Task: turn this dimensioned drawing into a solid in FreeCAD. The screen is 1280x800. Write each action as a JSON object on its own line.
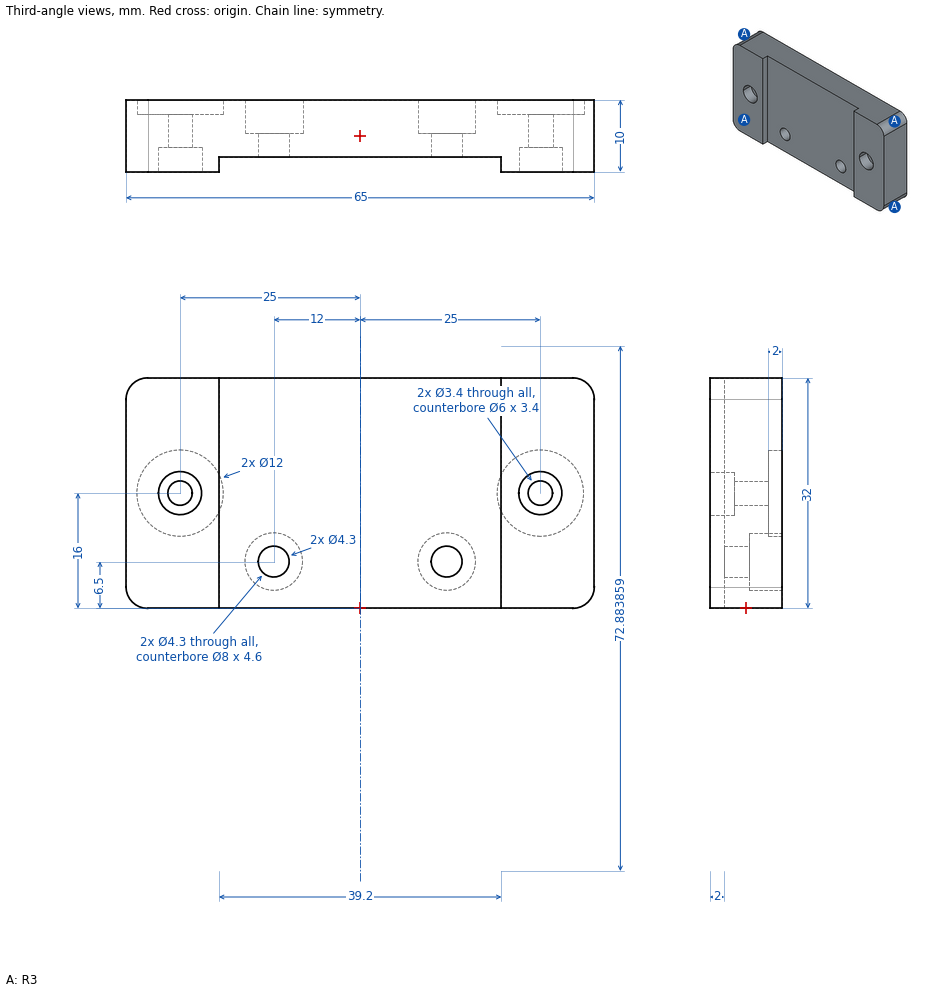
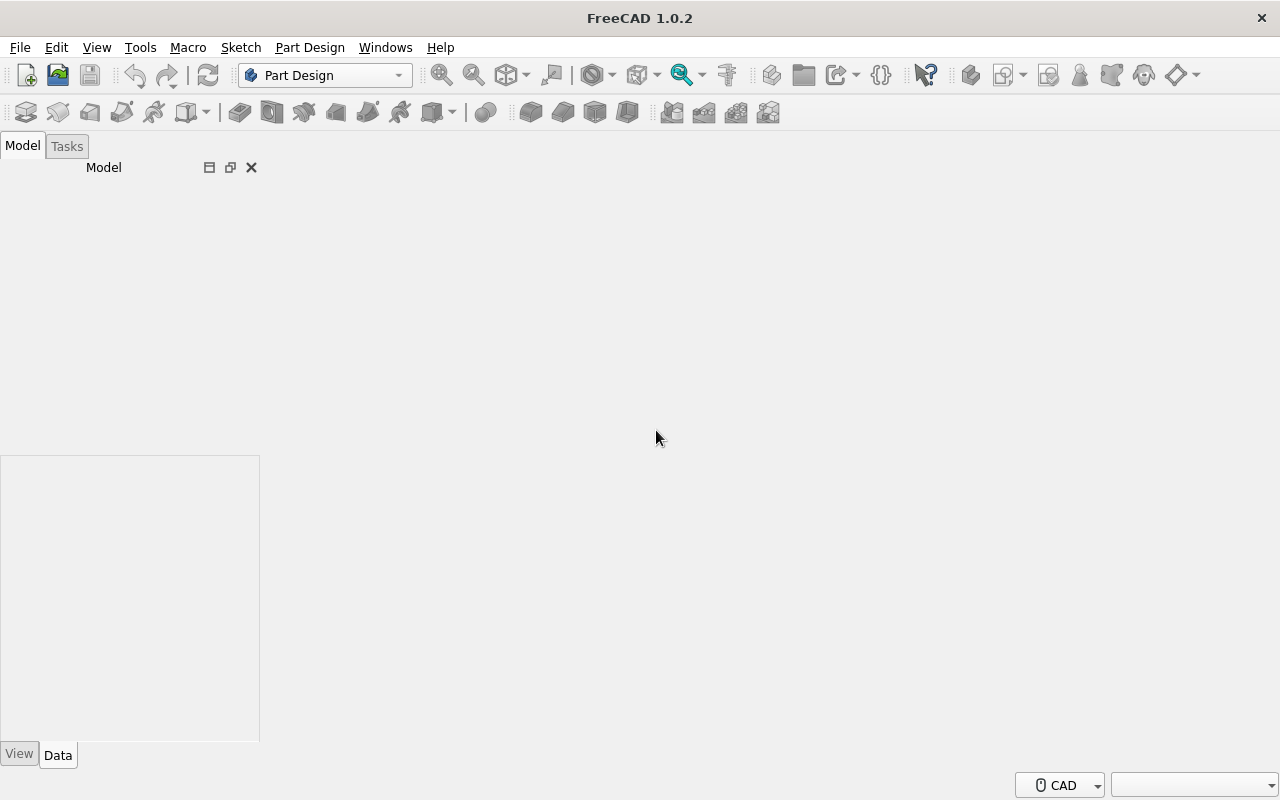
{"action": "left_click", "coordinate": [26, 76]}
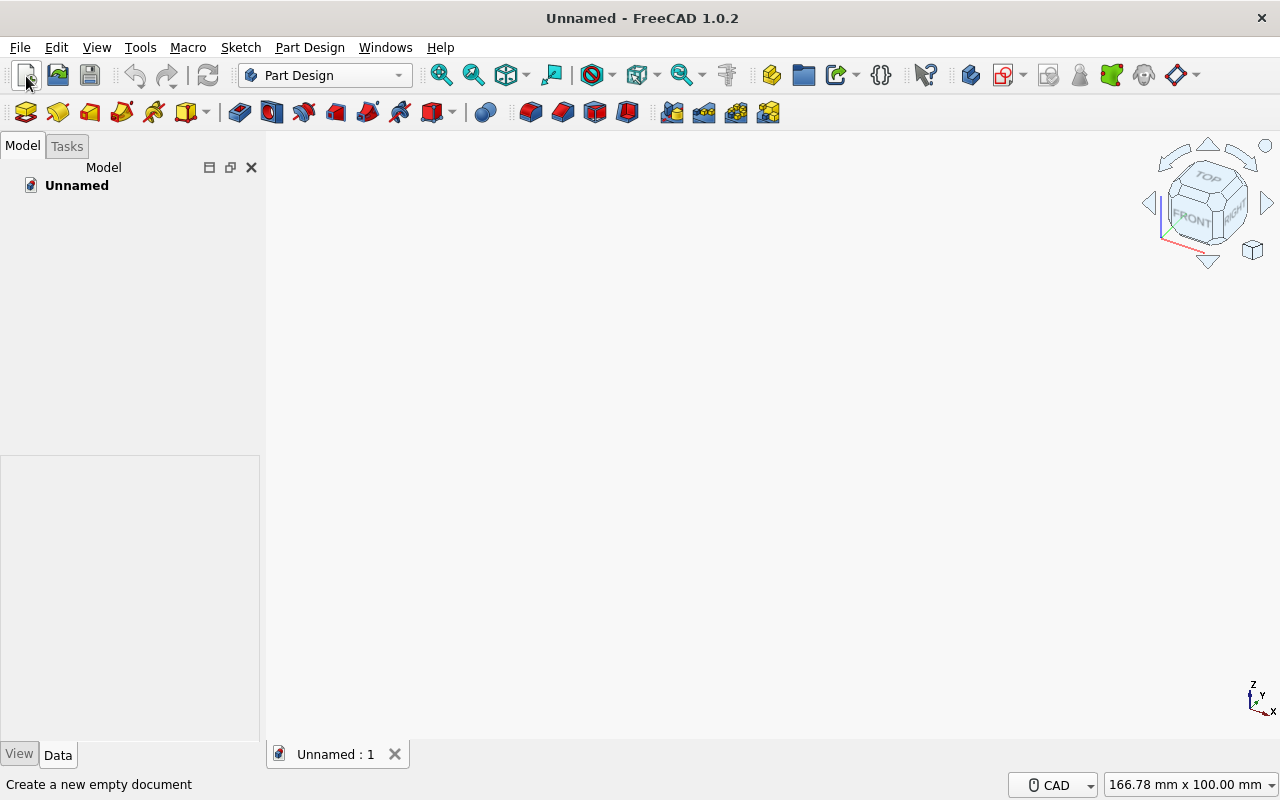
{"action": "left_click", "coordinate": [1004, 76]}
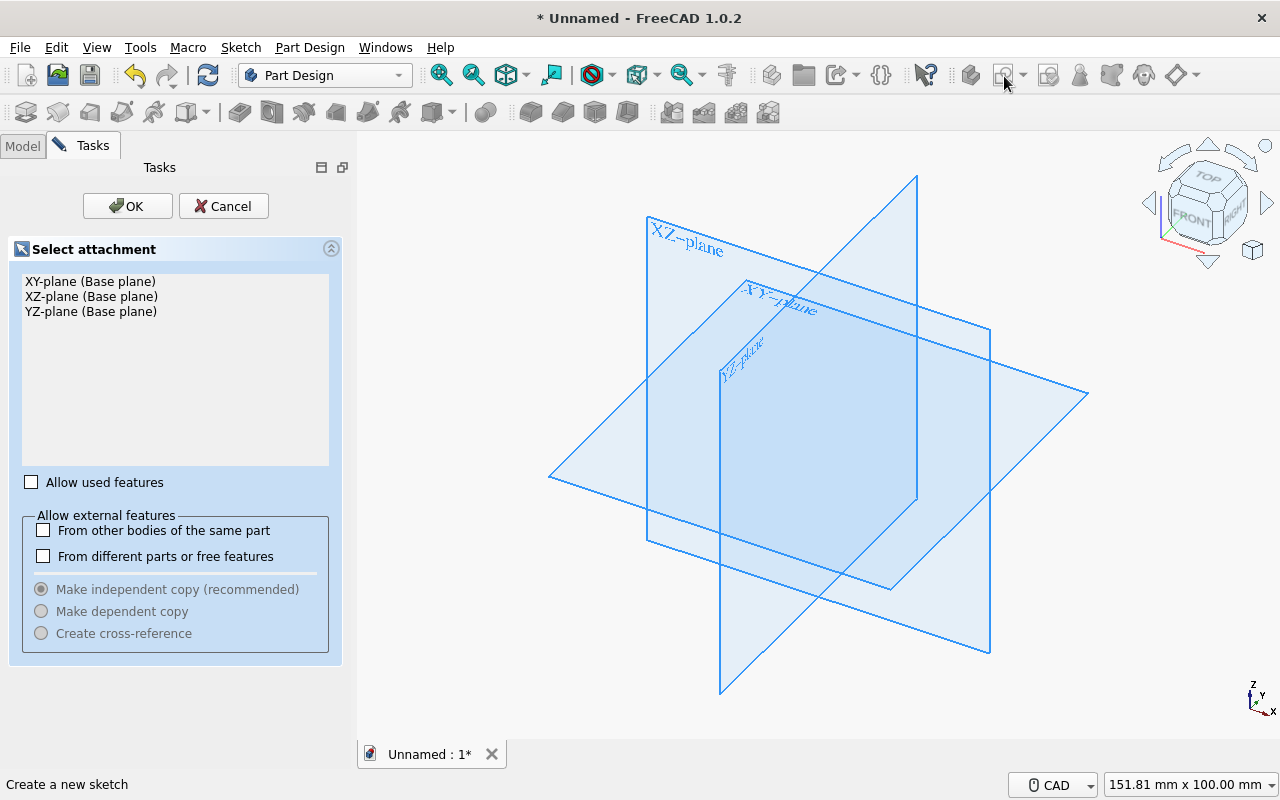
{"action": "left_click", "coordinate": [82, 282]}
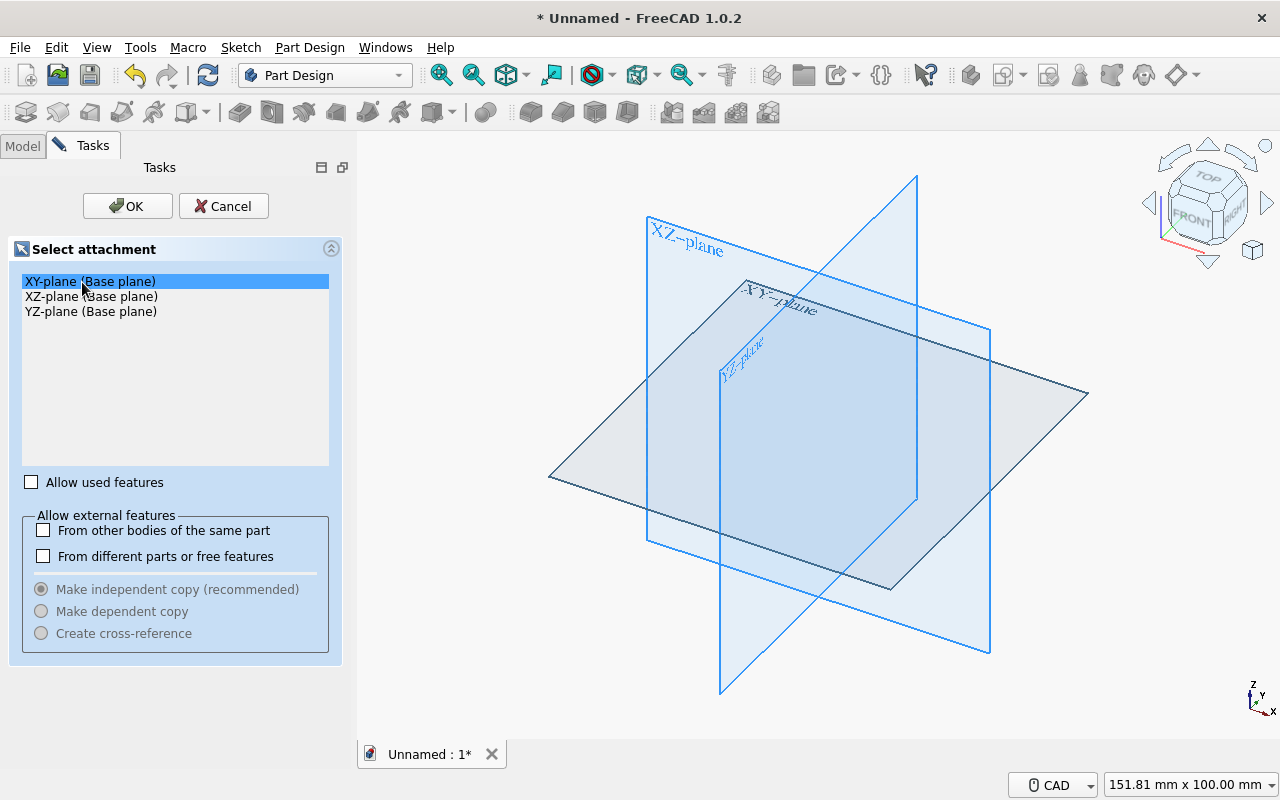
{"action": "left_click", "coordinate": [128, 206]}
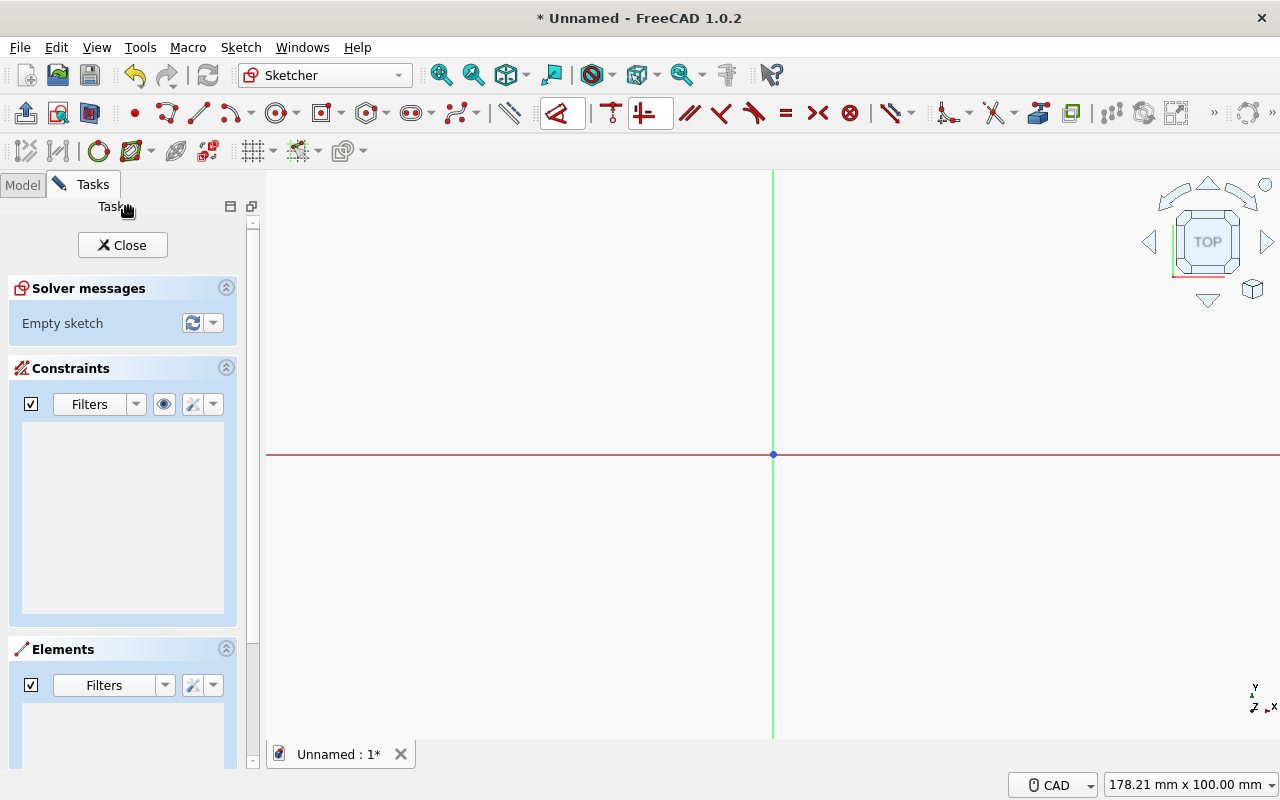
{"action": "scroll", "coordinate": [912, 455], "scroll_direction": "up", "scroll_amount": 2}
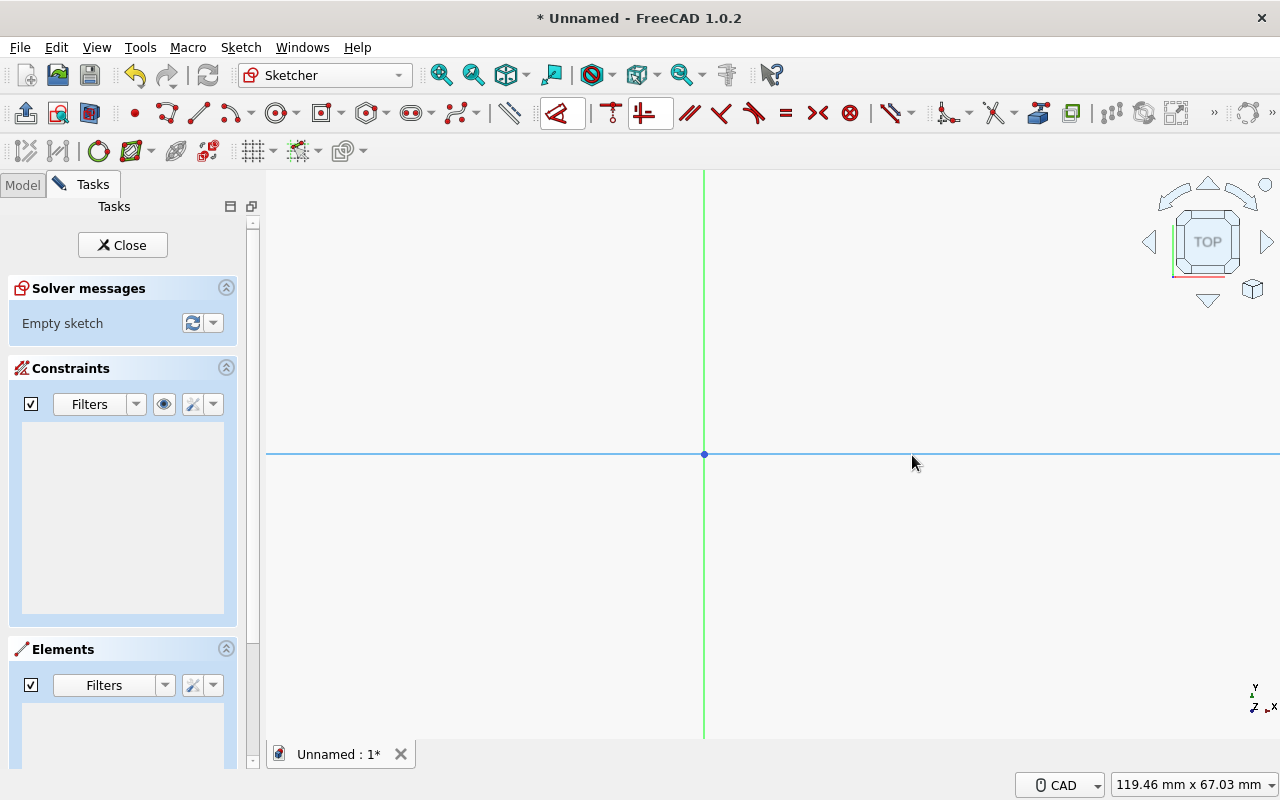
{"action": "left_click", "coordinate": [322, 114]}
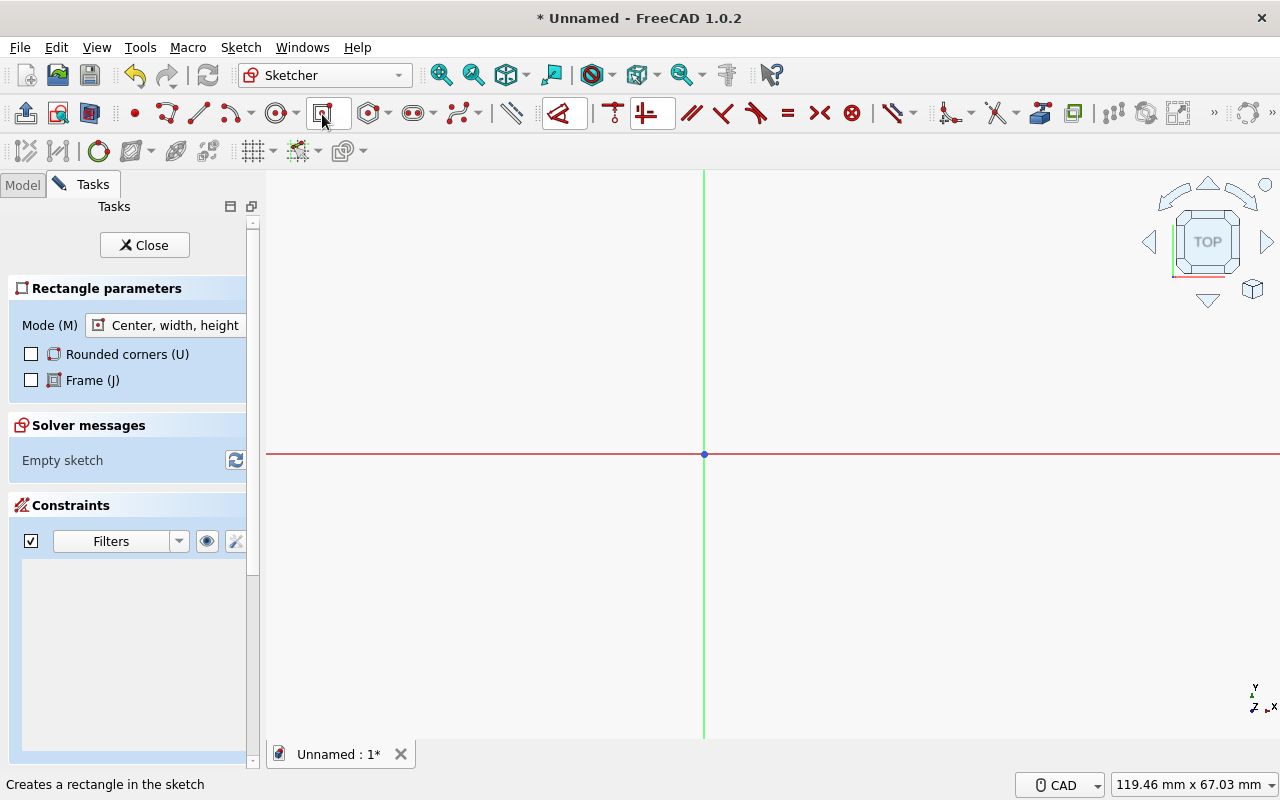
{"action": "left_click", "coordinate": [704, 454]}
{"action": "left_click", "coordinate": [980, 412]}
{"action": "key", "text": "Escape"}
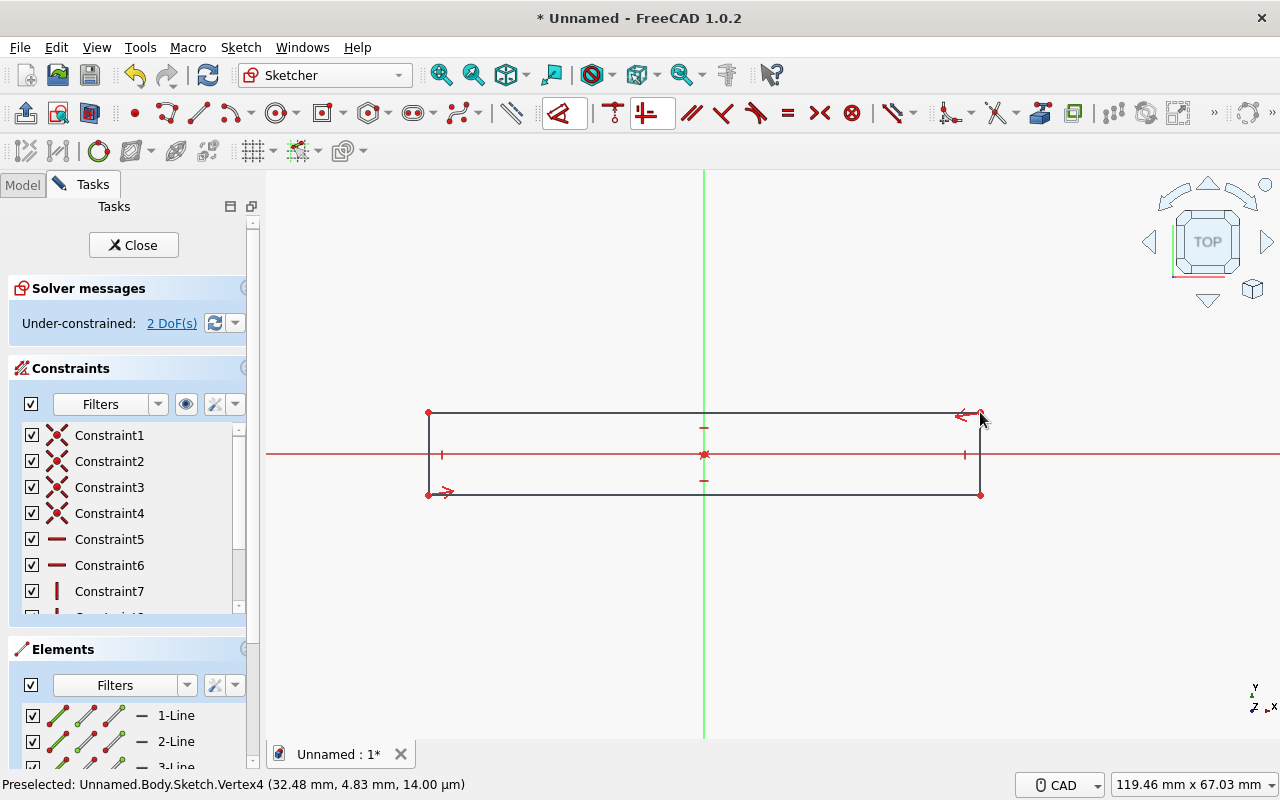
{"action": "left_click", "coordinate": [594, 495]}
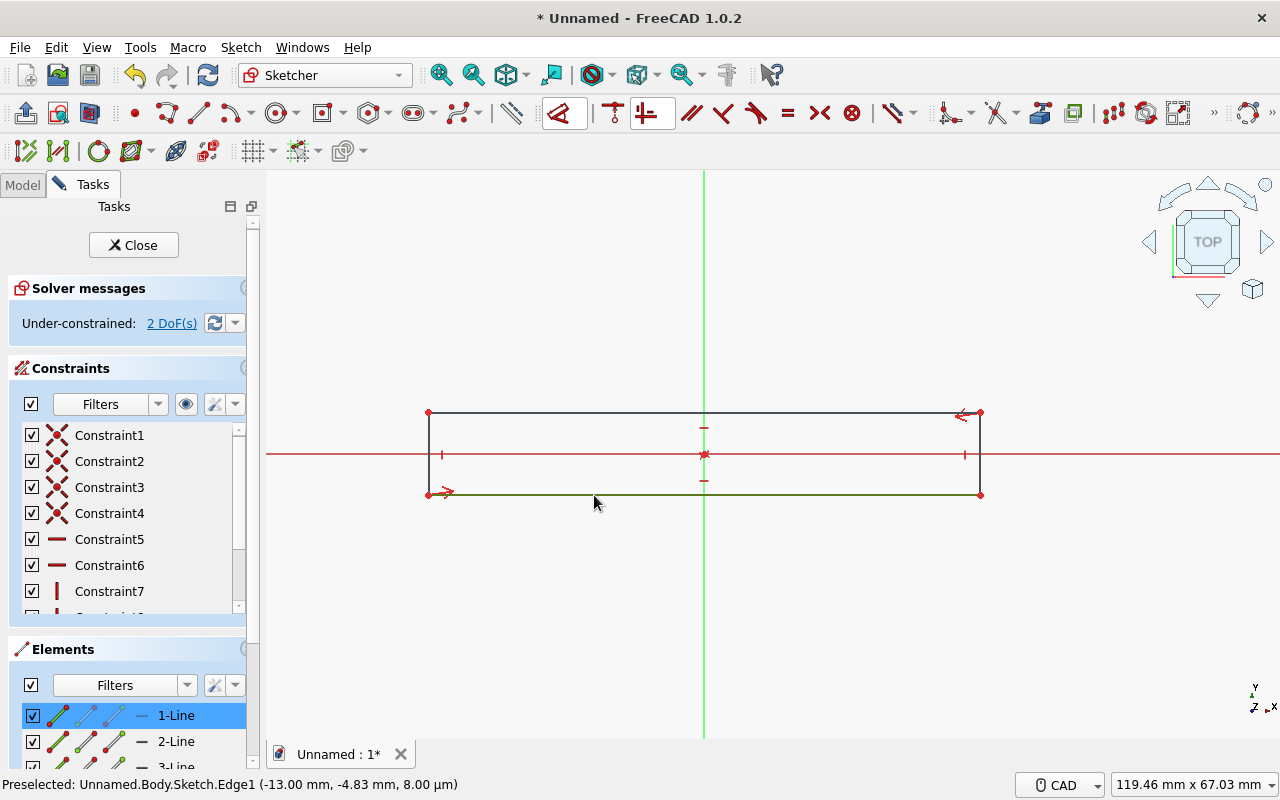
{"action": "left_click", "coordinate": [582, 114]}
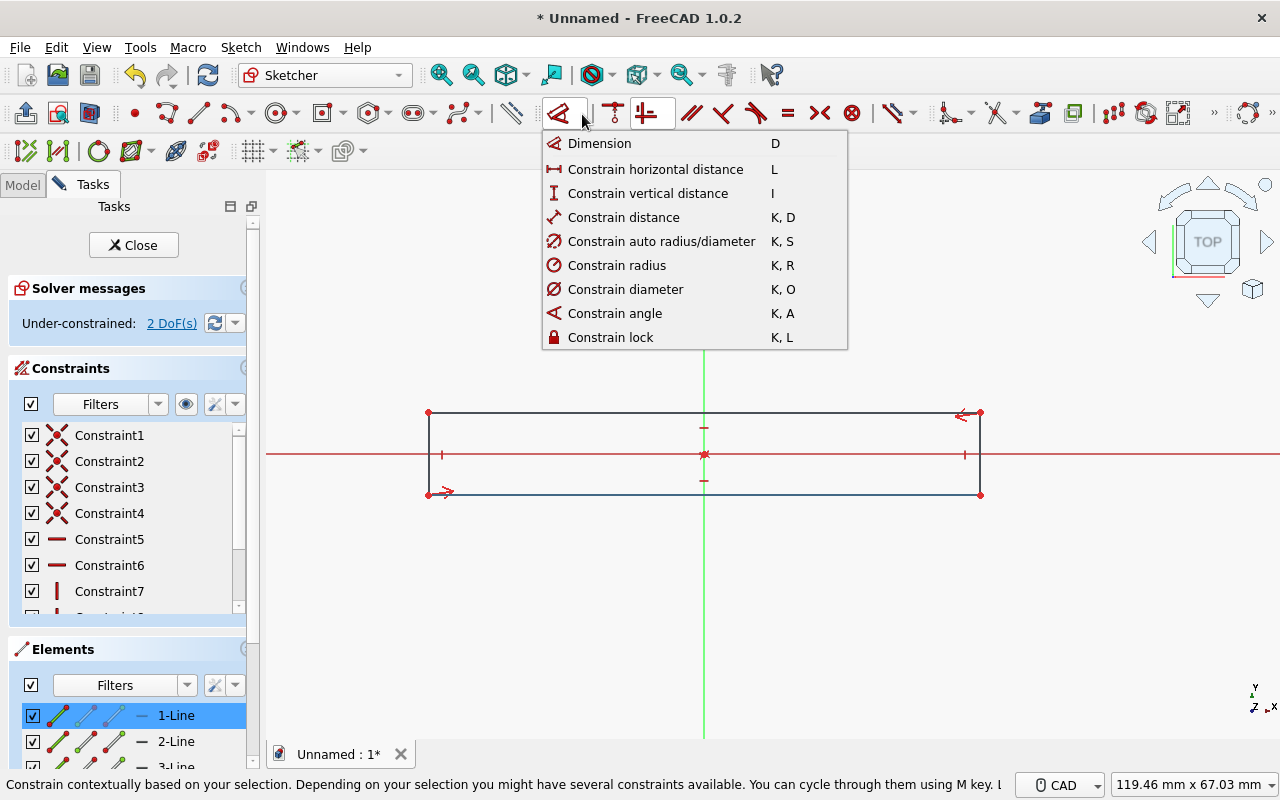
{"action": "left_click", "coordinate": [695, 169]}